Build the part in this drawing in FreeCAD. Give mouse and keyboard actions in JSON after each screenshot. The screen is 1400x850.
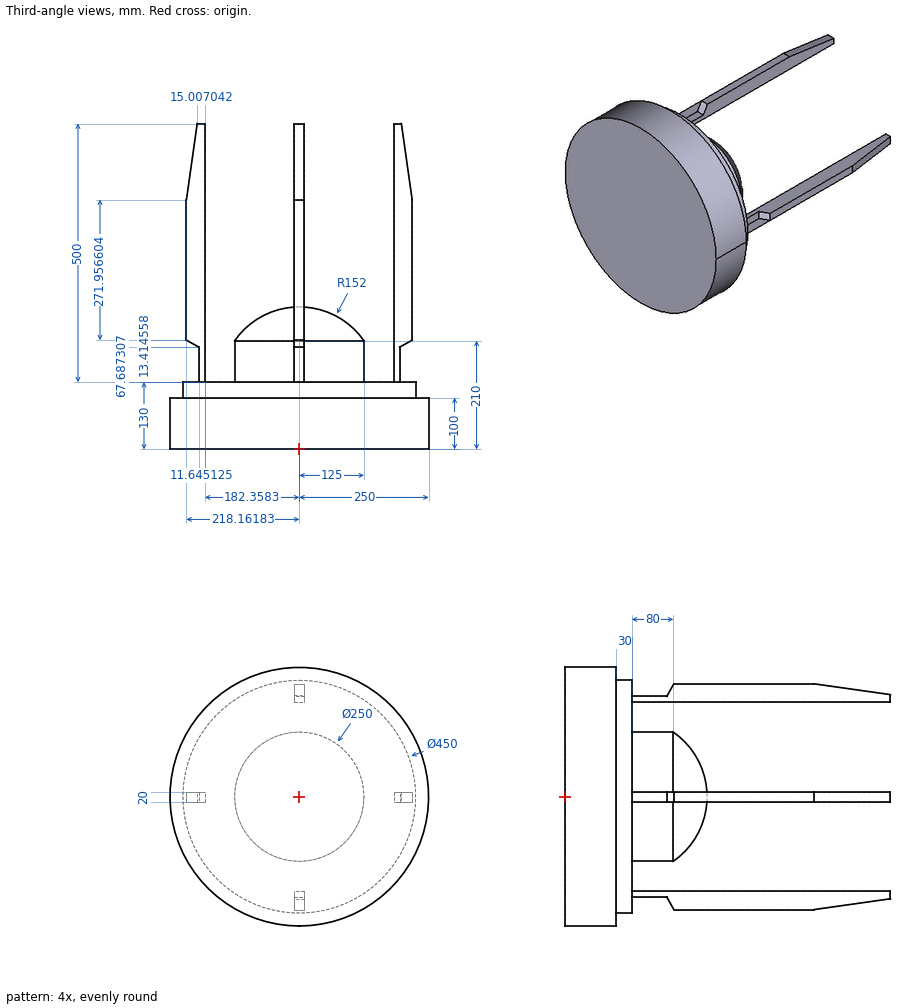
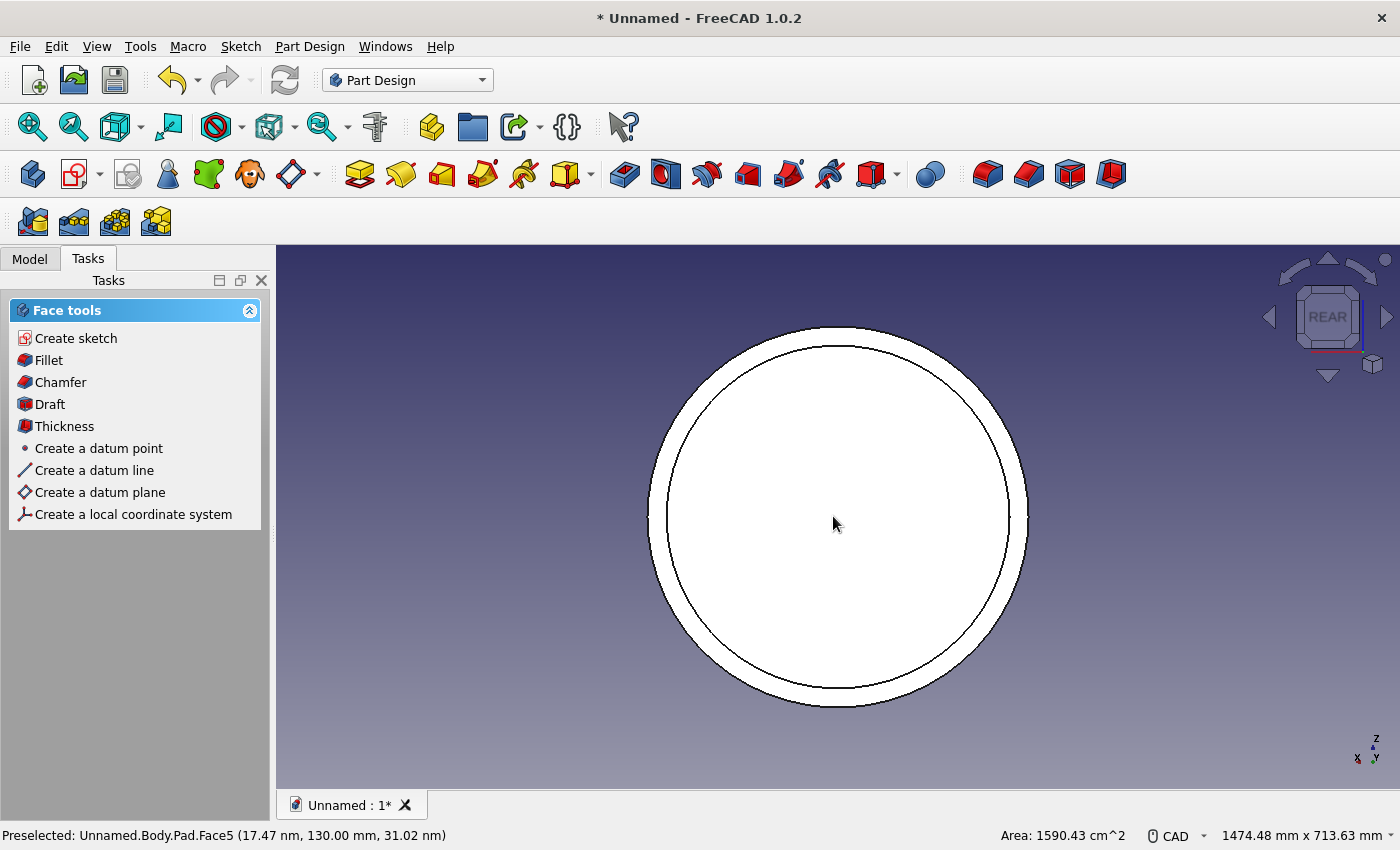
{"action": "left_click", "coordinate": [74, 174]}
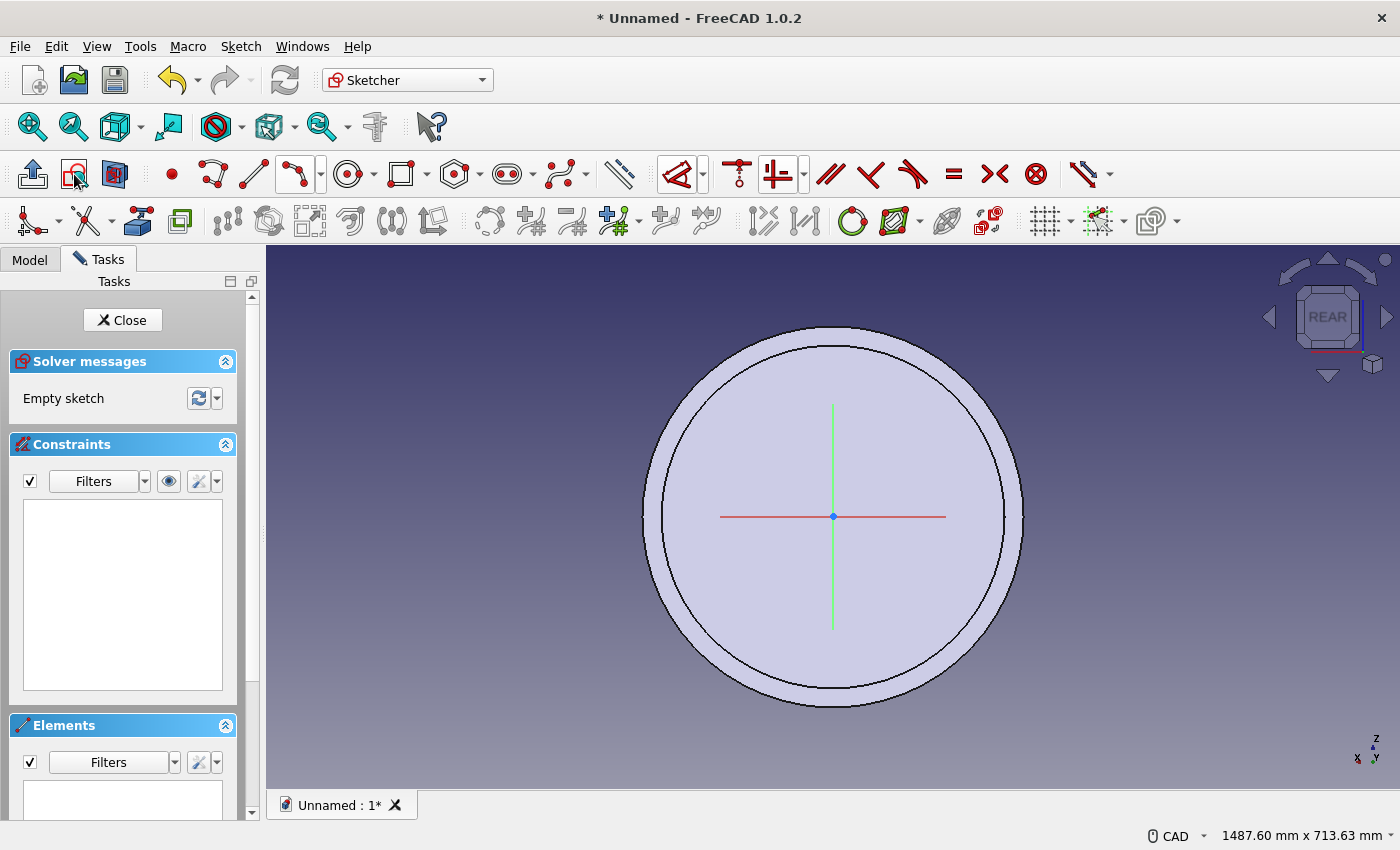
{"action": "scroll", "coordinate": [916, 517], "scroll_direction": "up", "scroll_amount": 3}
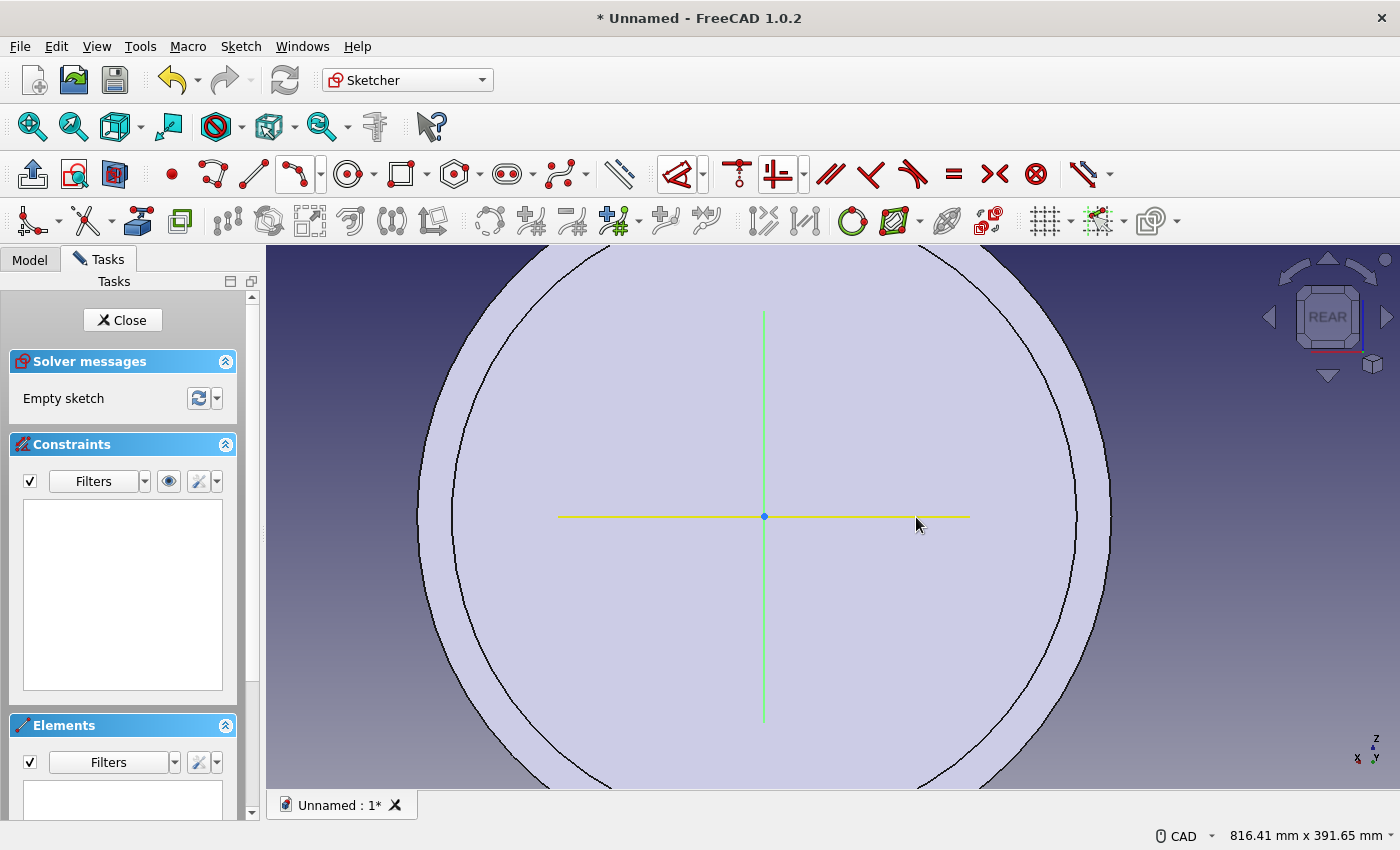
{"action": "left_click", "coordinate": [348, 174]}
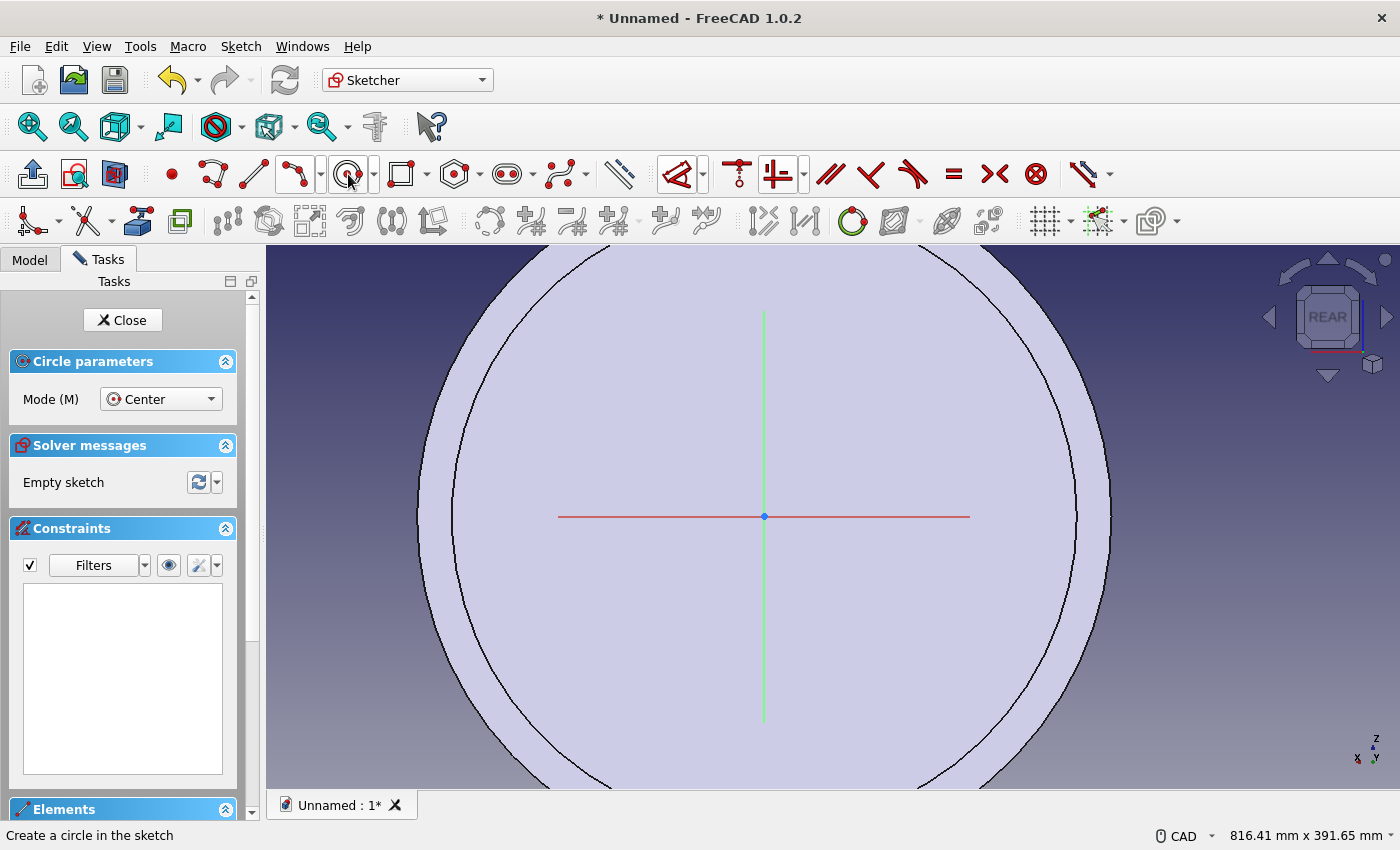
{"action": "left_click", "coordinate": [764, 517]}
{"action": "left_click", "coordinate": [887, 394]}
{"action": "key", "text": "Escape"}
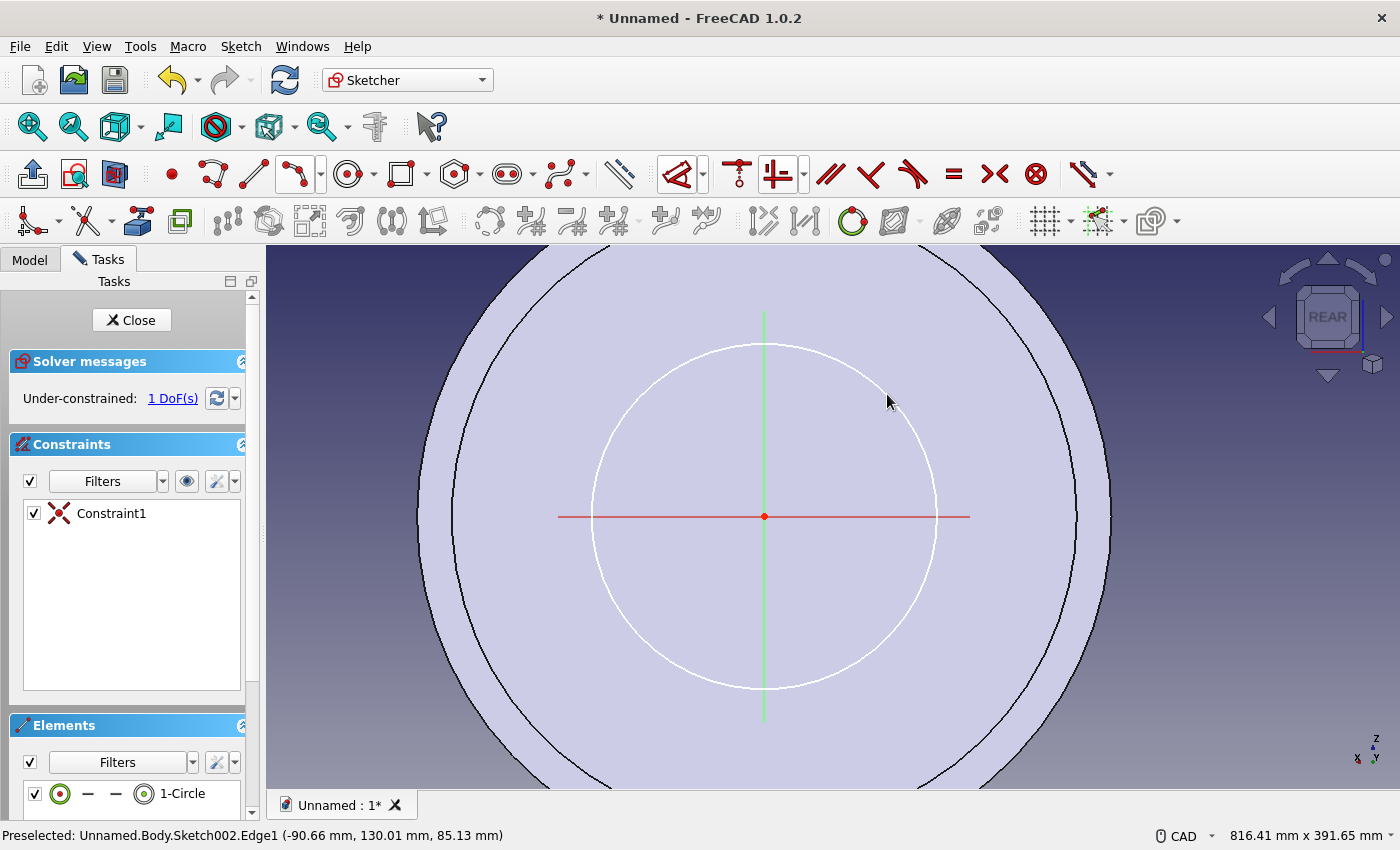
{"action": "left_click", "coordinate": [886, 394]}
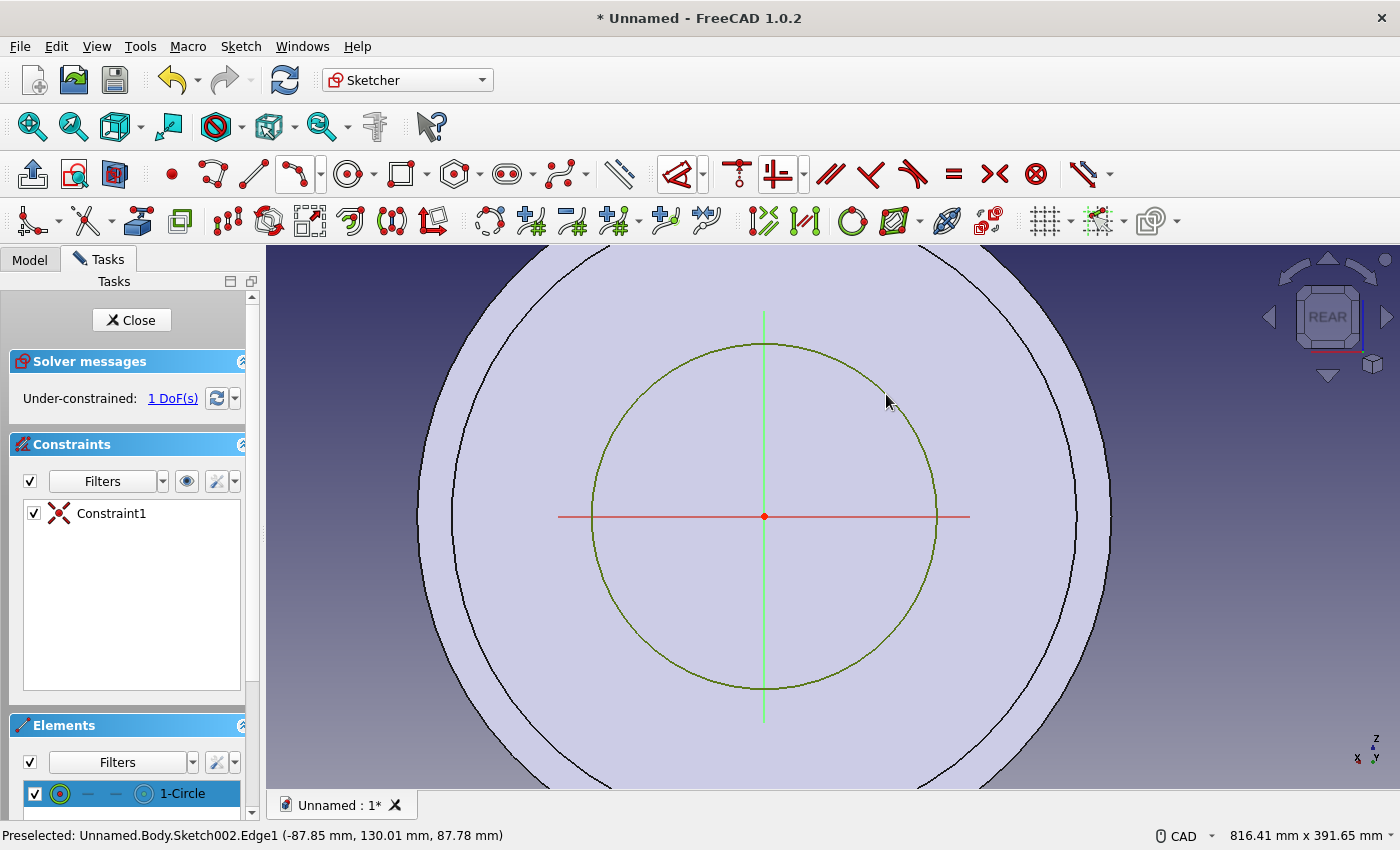
{"action": "left_click", "coordinate": [702, 174]}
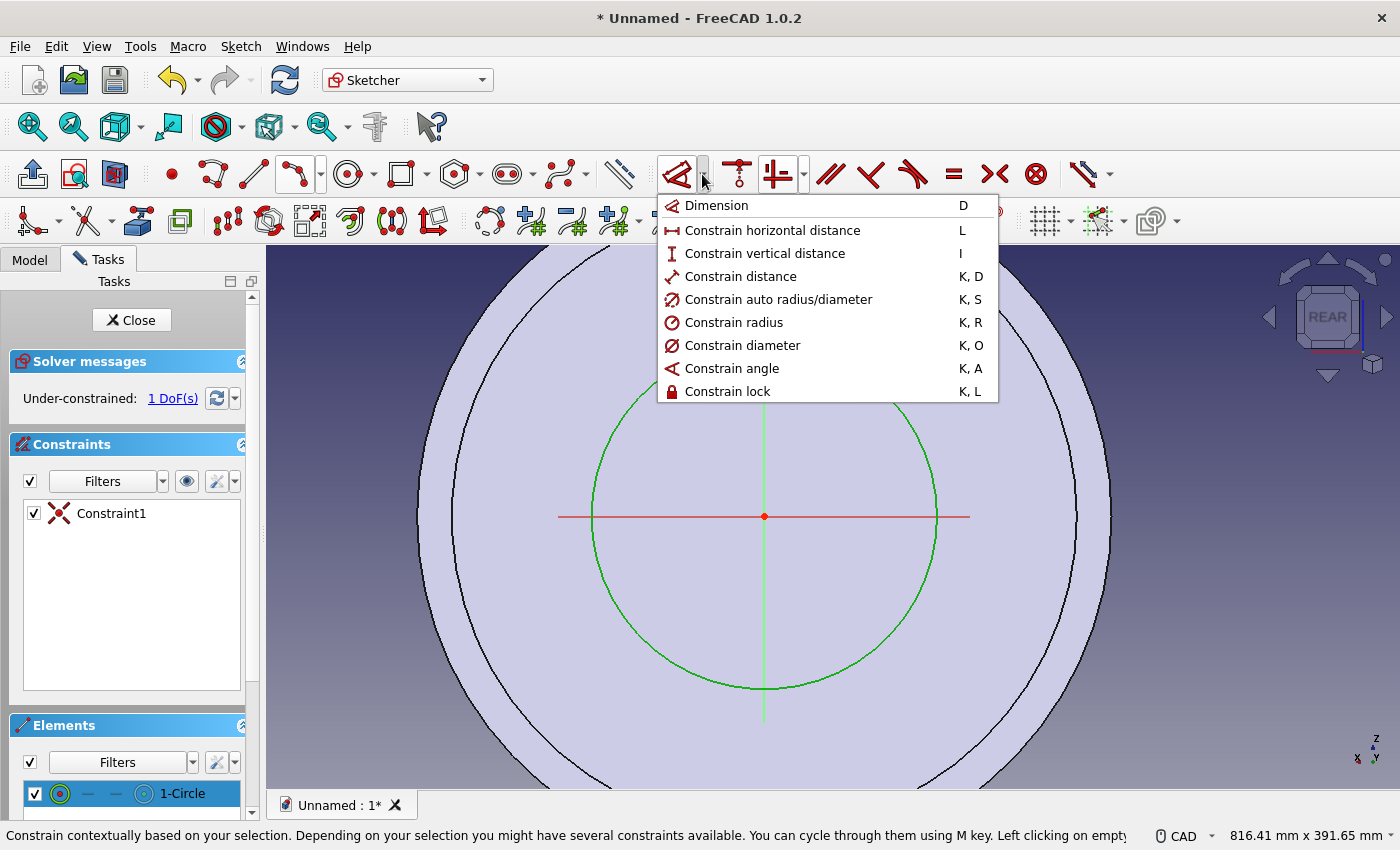
{"action": "left_click", "coordinate": [828, 346]}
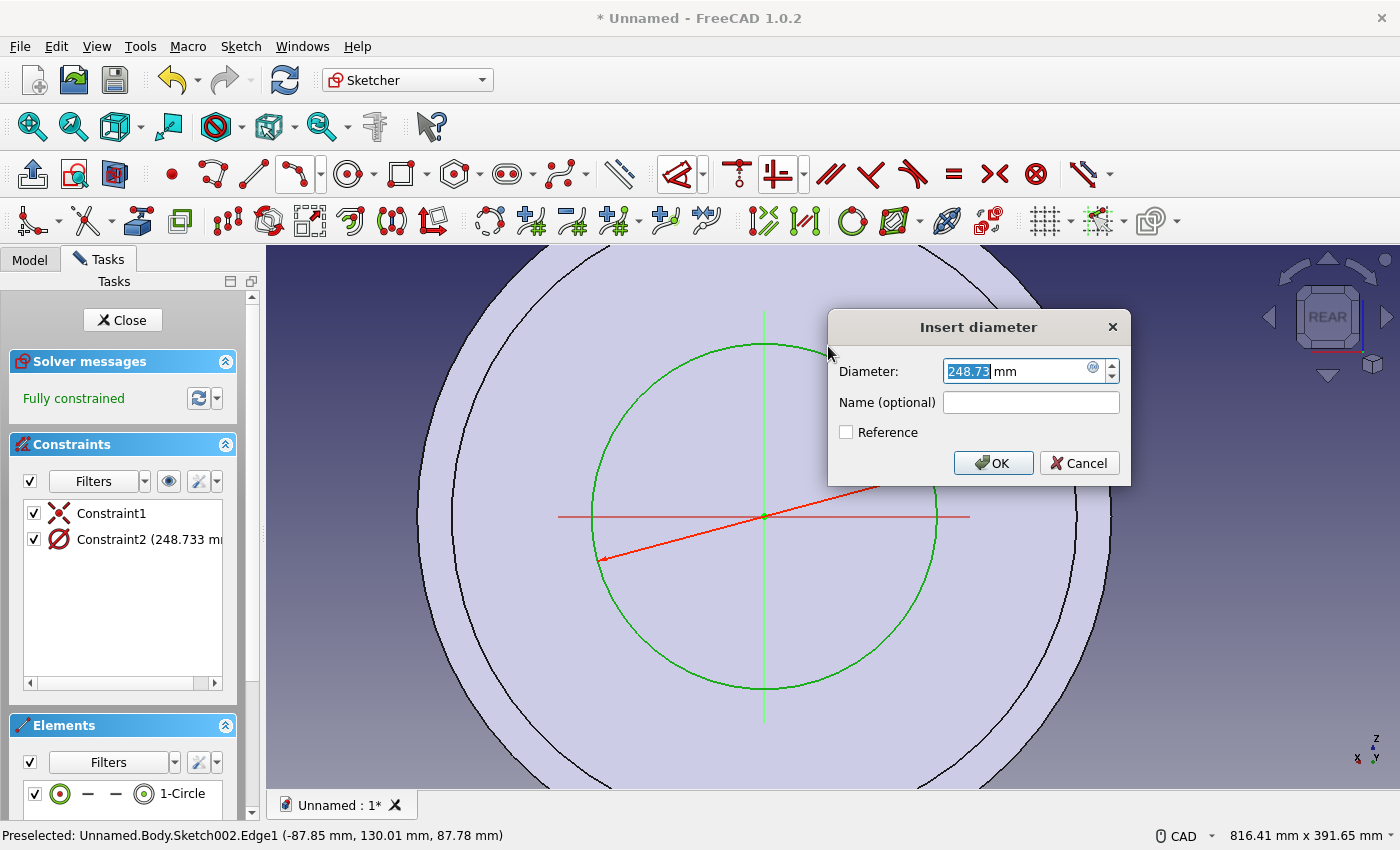
{"action": "type", "text": "250"}
{"action": "key", "text": "Return"}